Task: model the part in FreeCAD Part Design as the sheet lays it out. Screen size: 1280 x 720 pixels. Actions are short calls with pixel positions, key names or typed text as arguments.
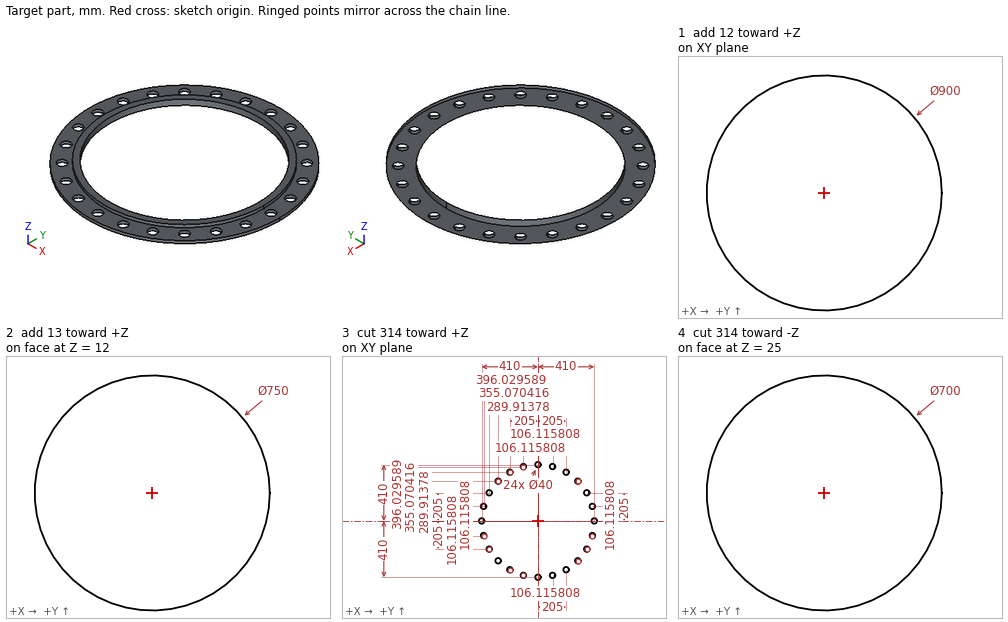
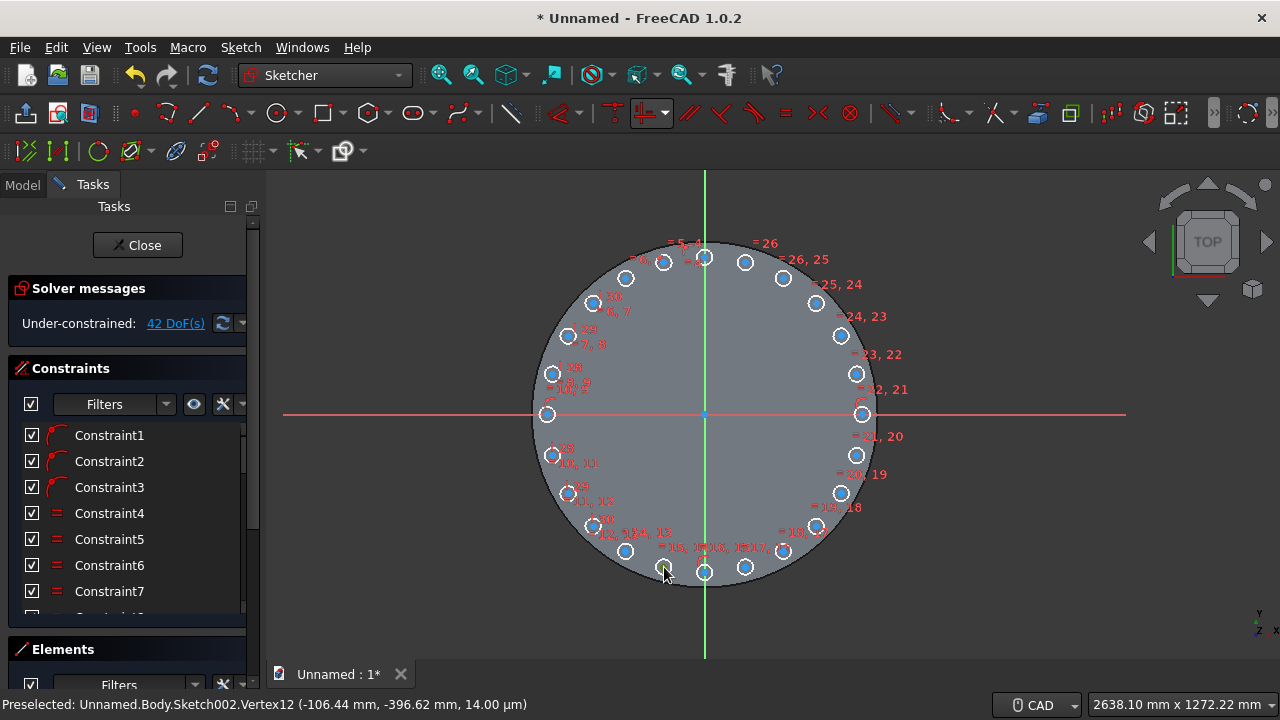
click(745, 567)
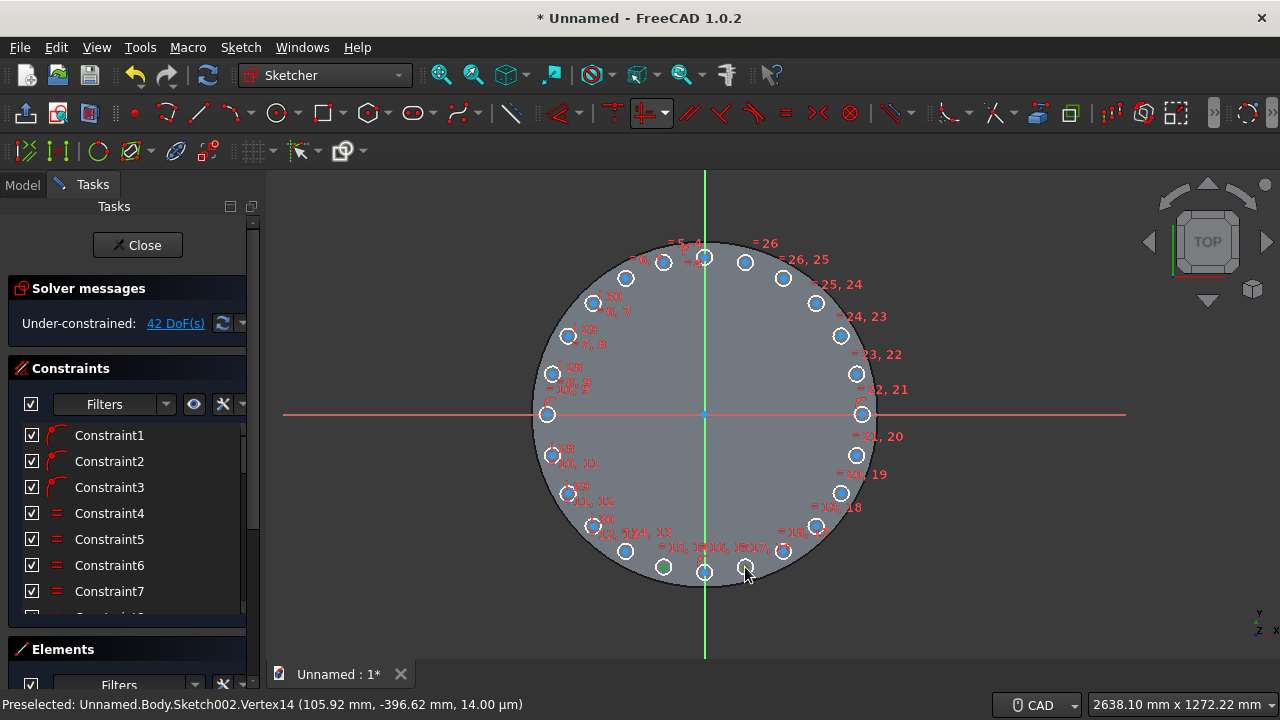
key(h)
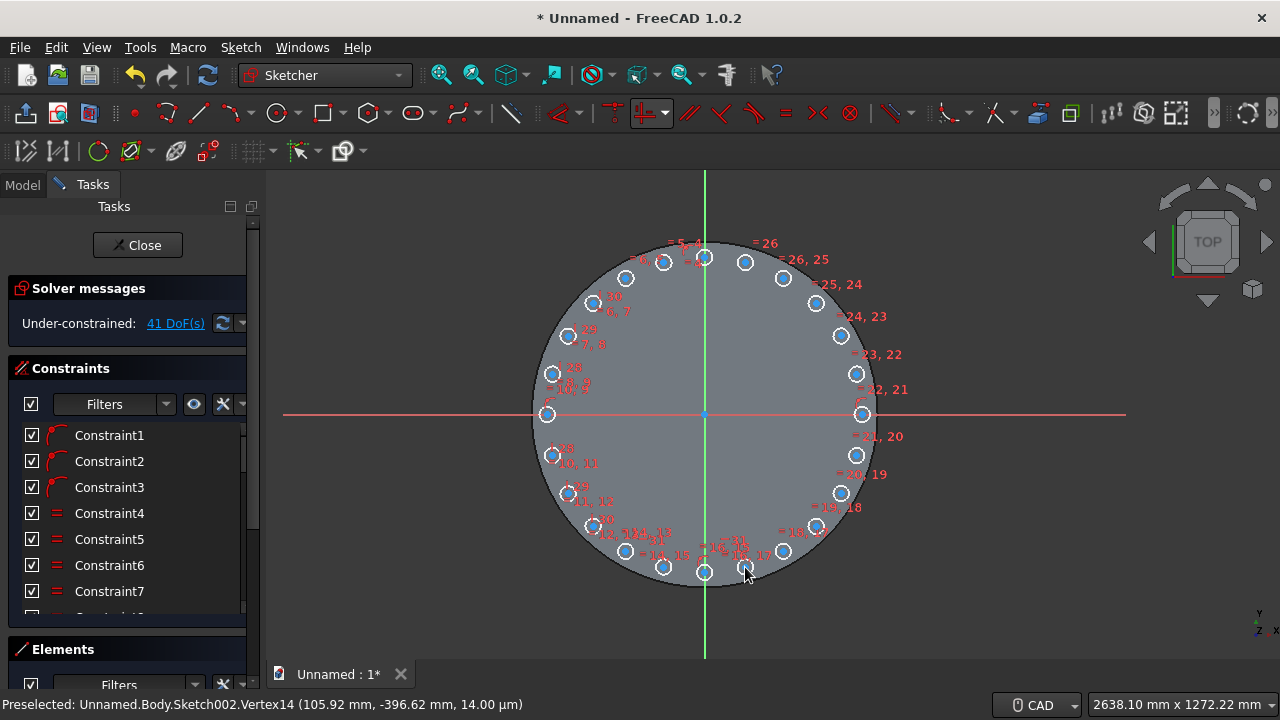
click(626, 551)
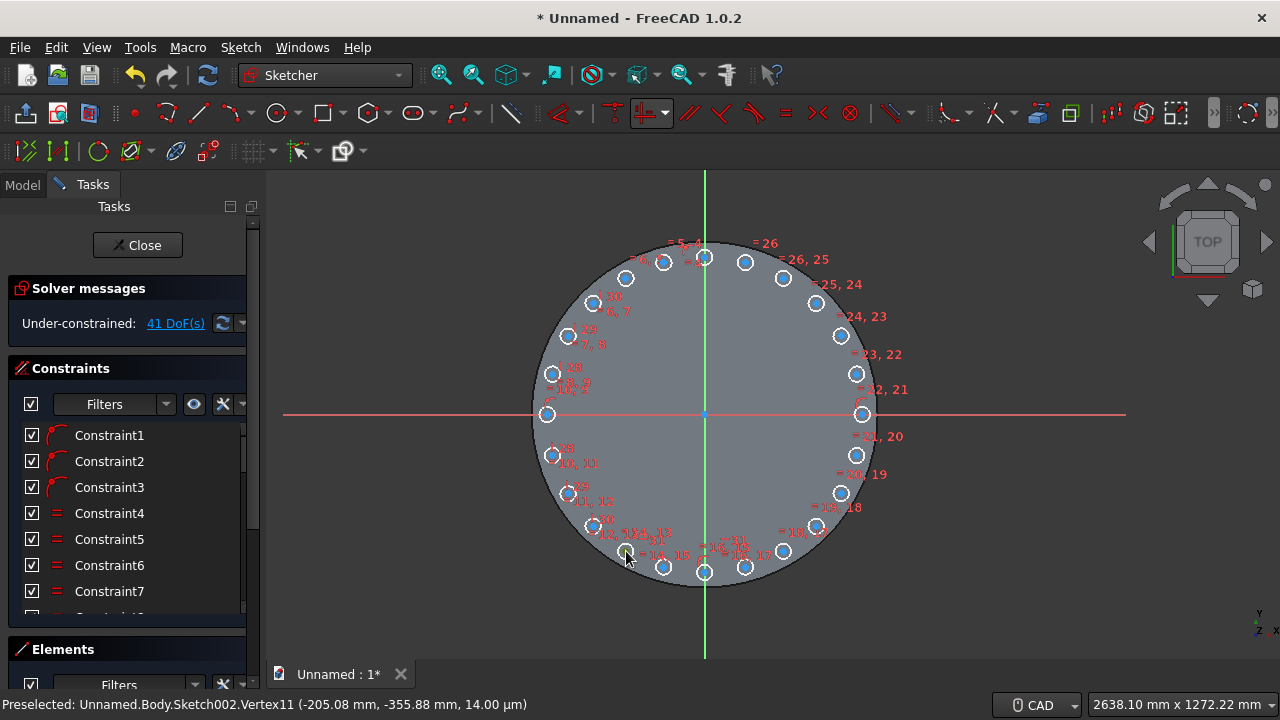
click(783, 551)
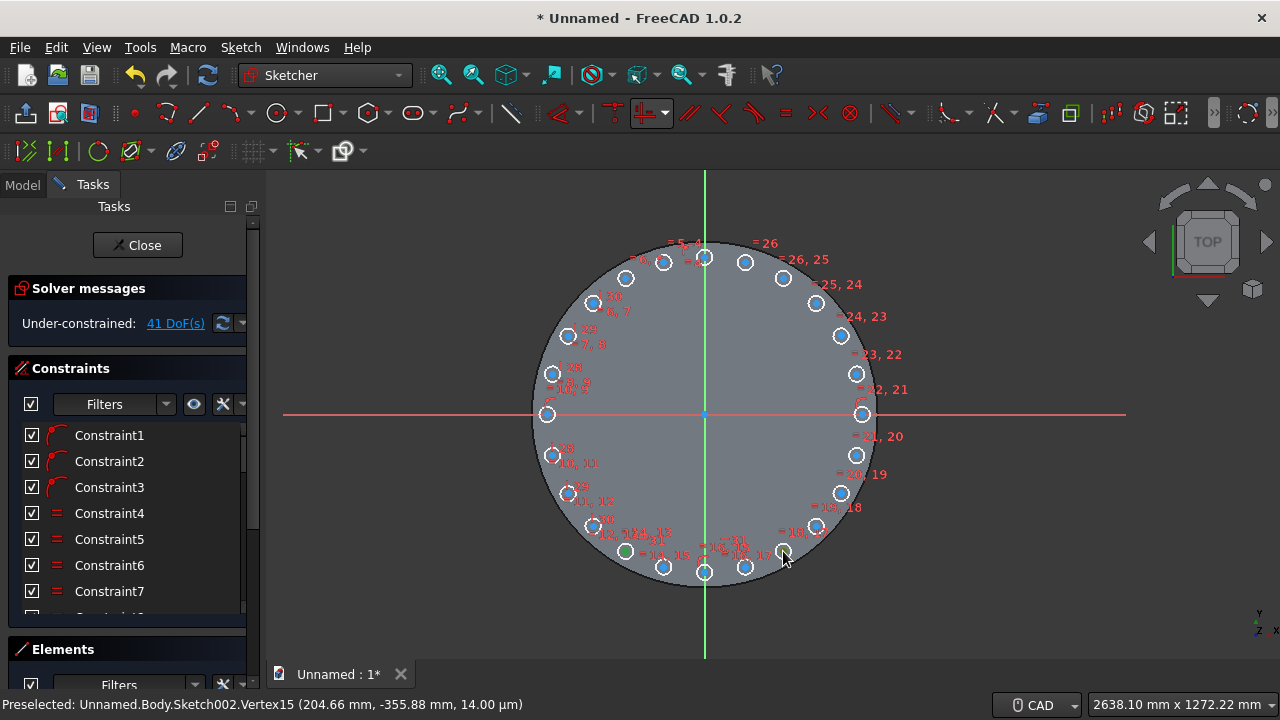
key(h)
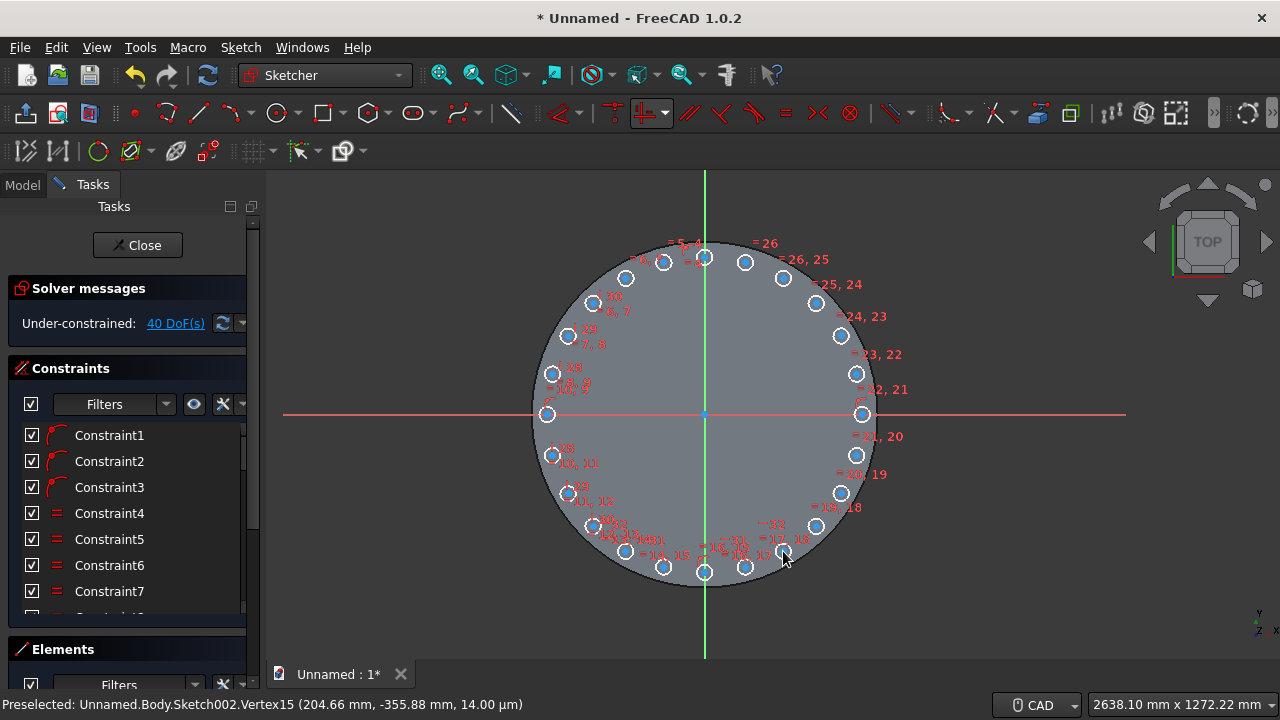
scroll(593, 526, up, 4)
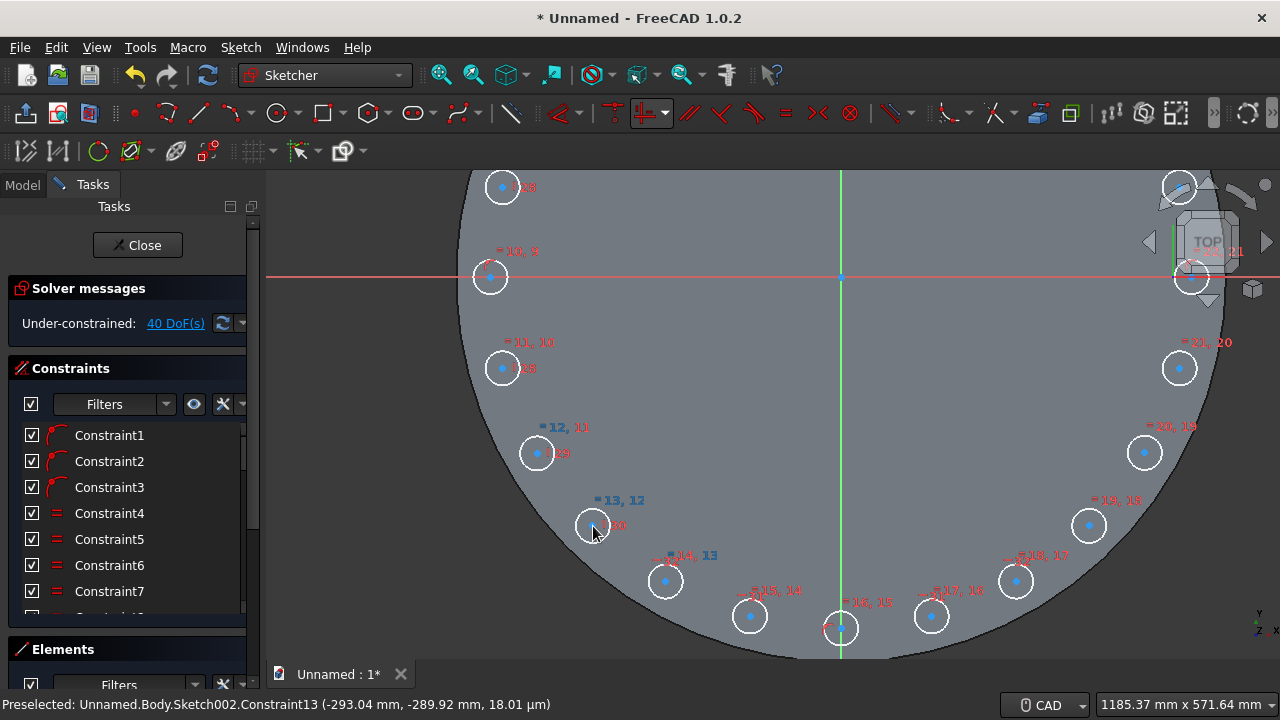
click(593, 526)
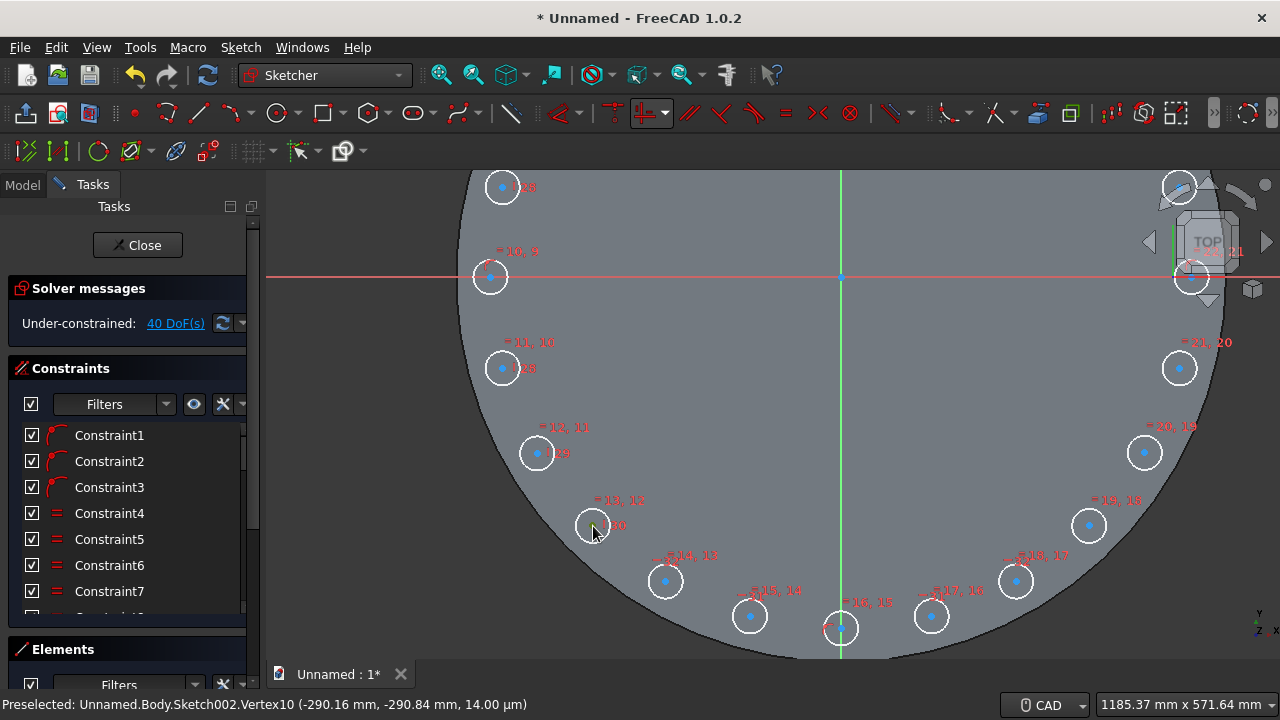
click(1089, 526)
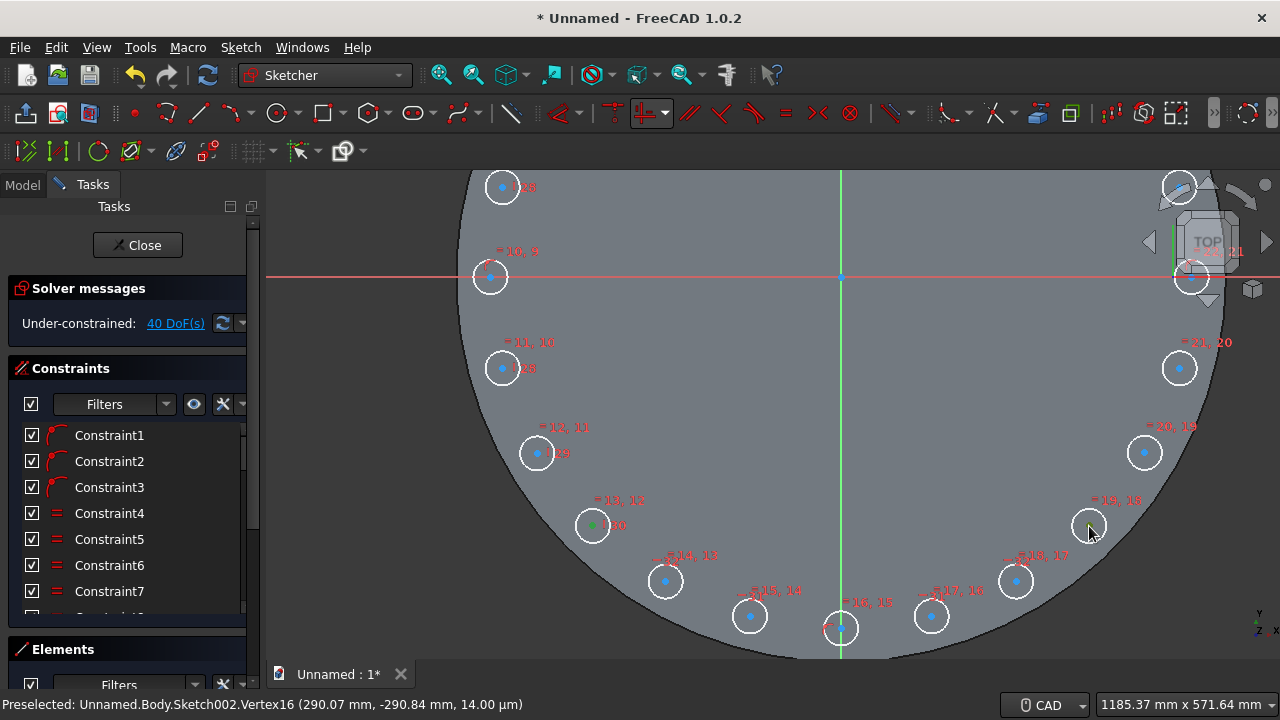
key(h)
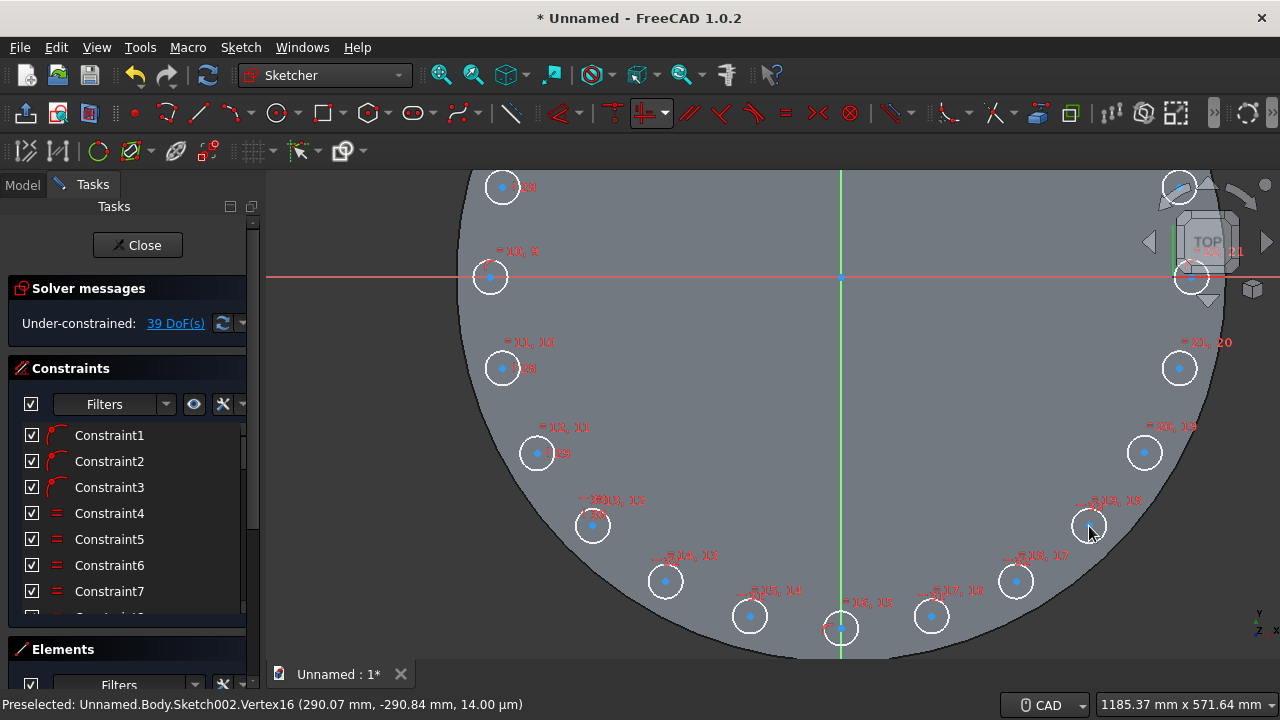
scroll(593, 527, down, 4)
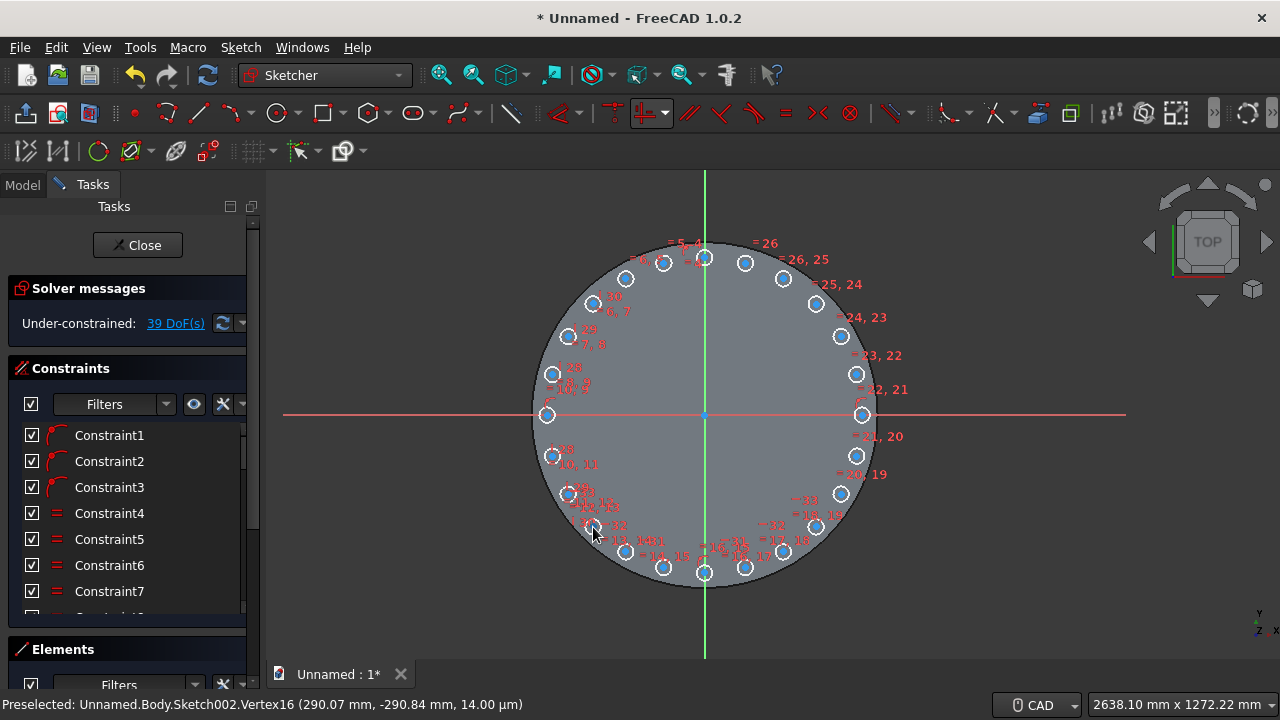
click(857, 456)